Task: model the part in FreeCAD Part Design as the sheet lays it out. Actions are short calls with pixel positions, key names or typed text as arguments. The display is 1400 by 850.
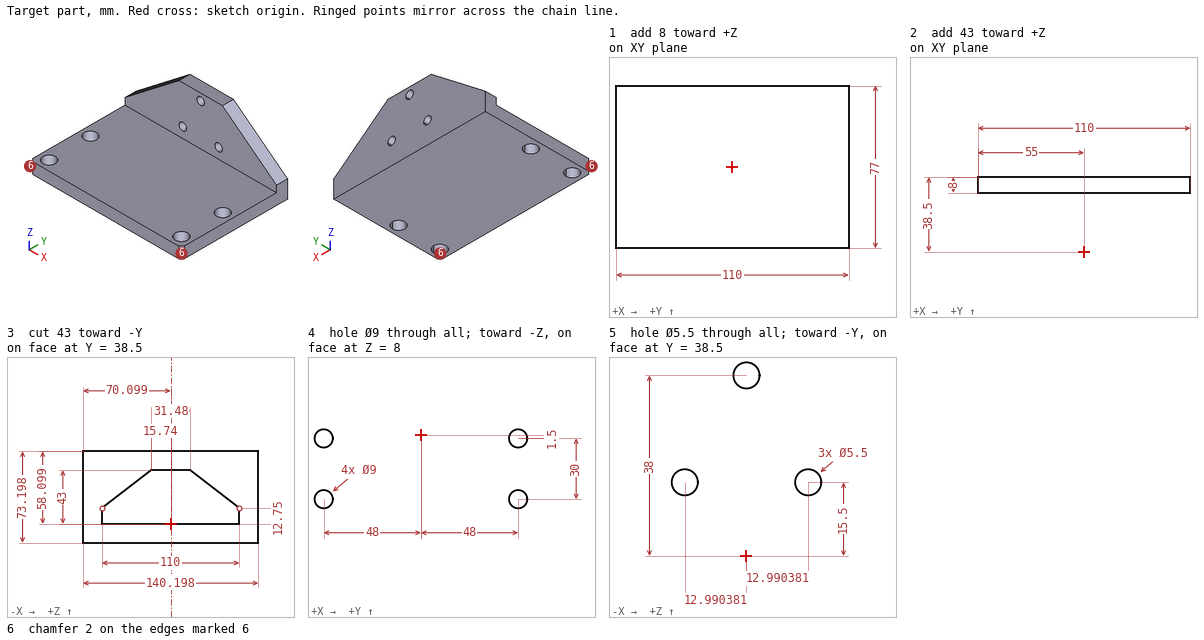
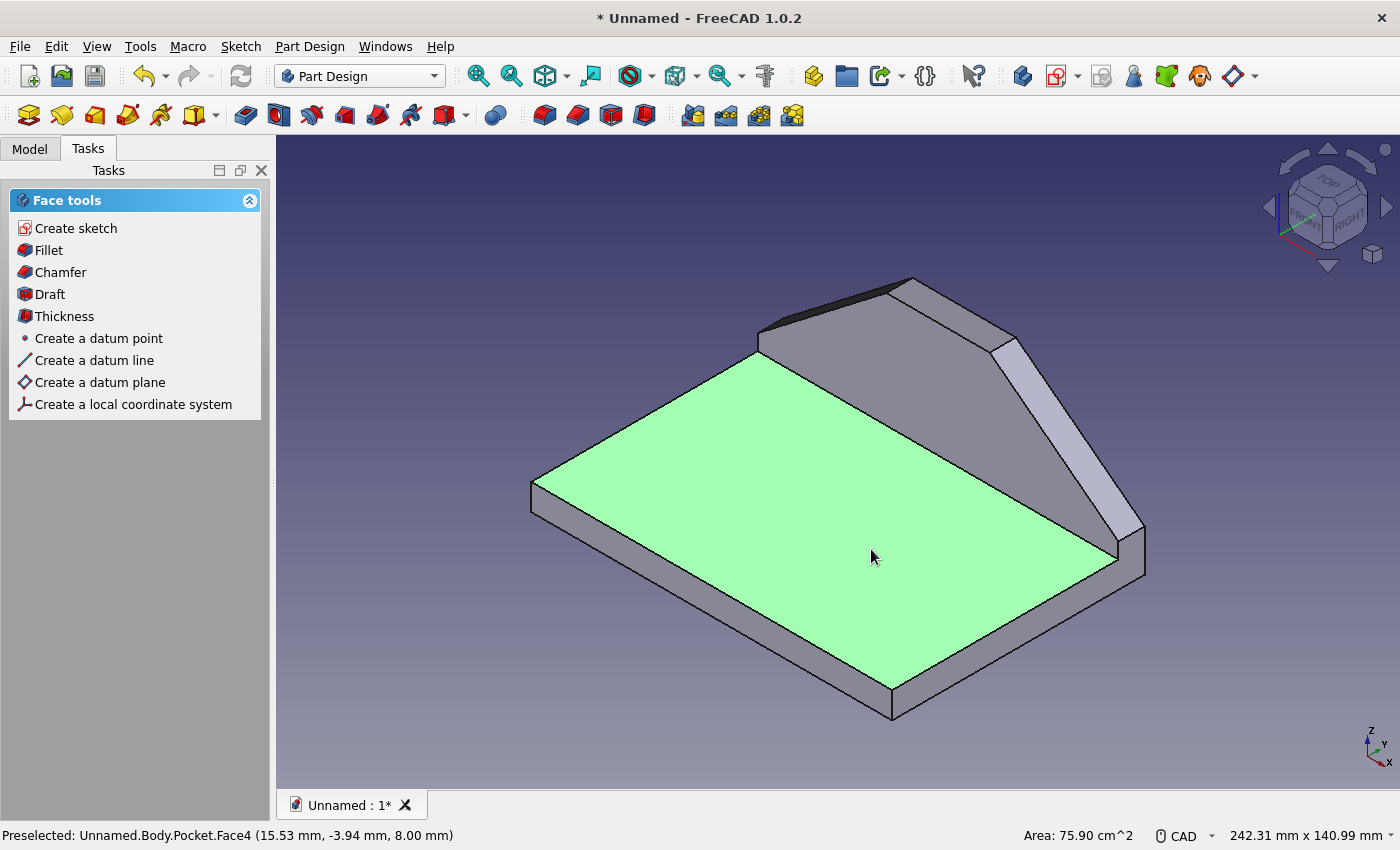
click(1056, 76)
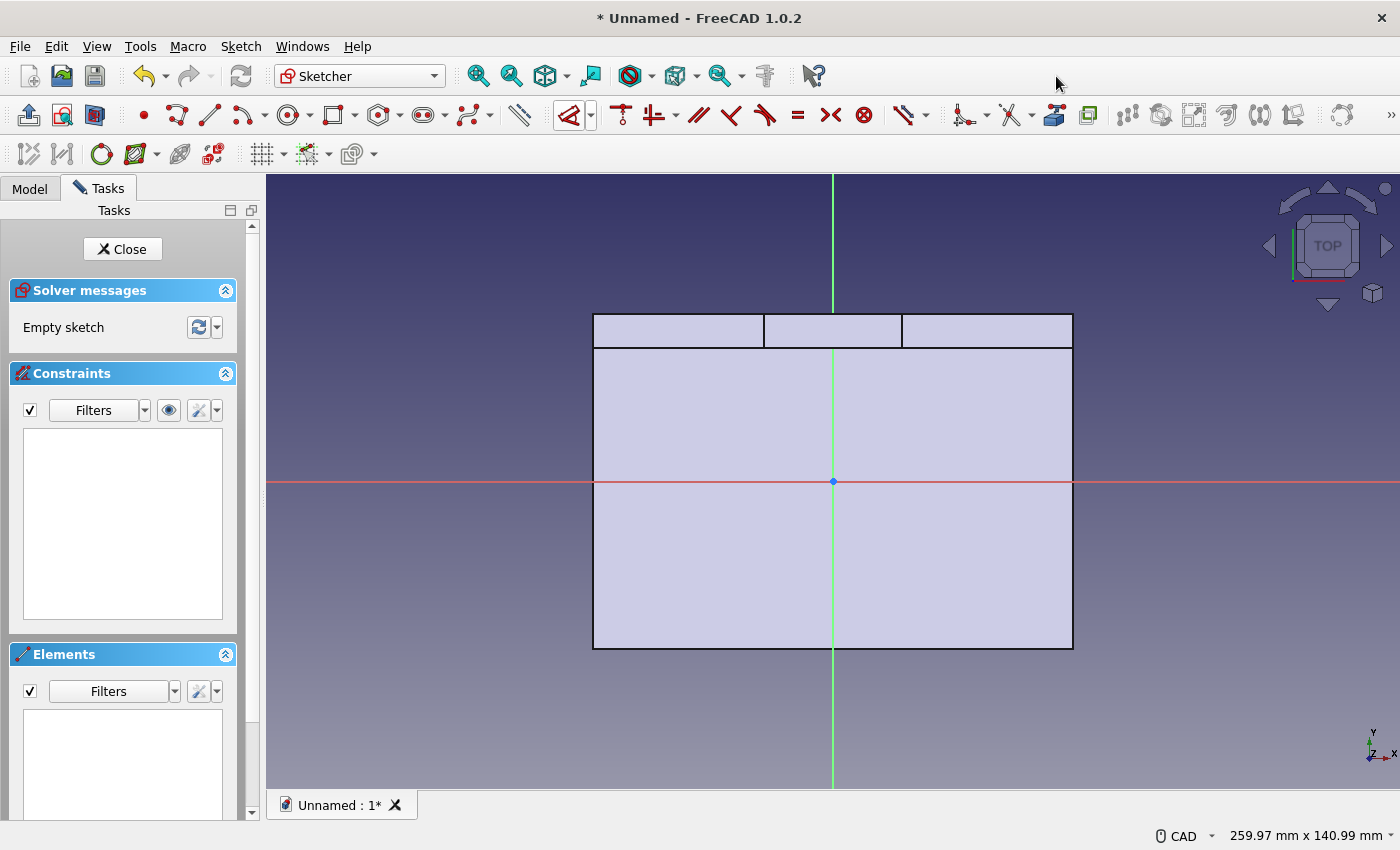
scroll(972, 700, up, 2)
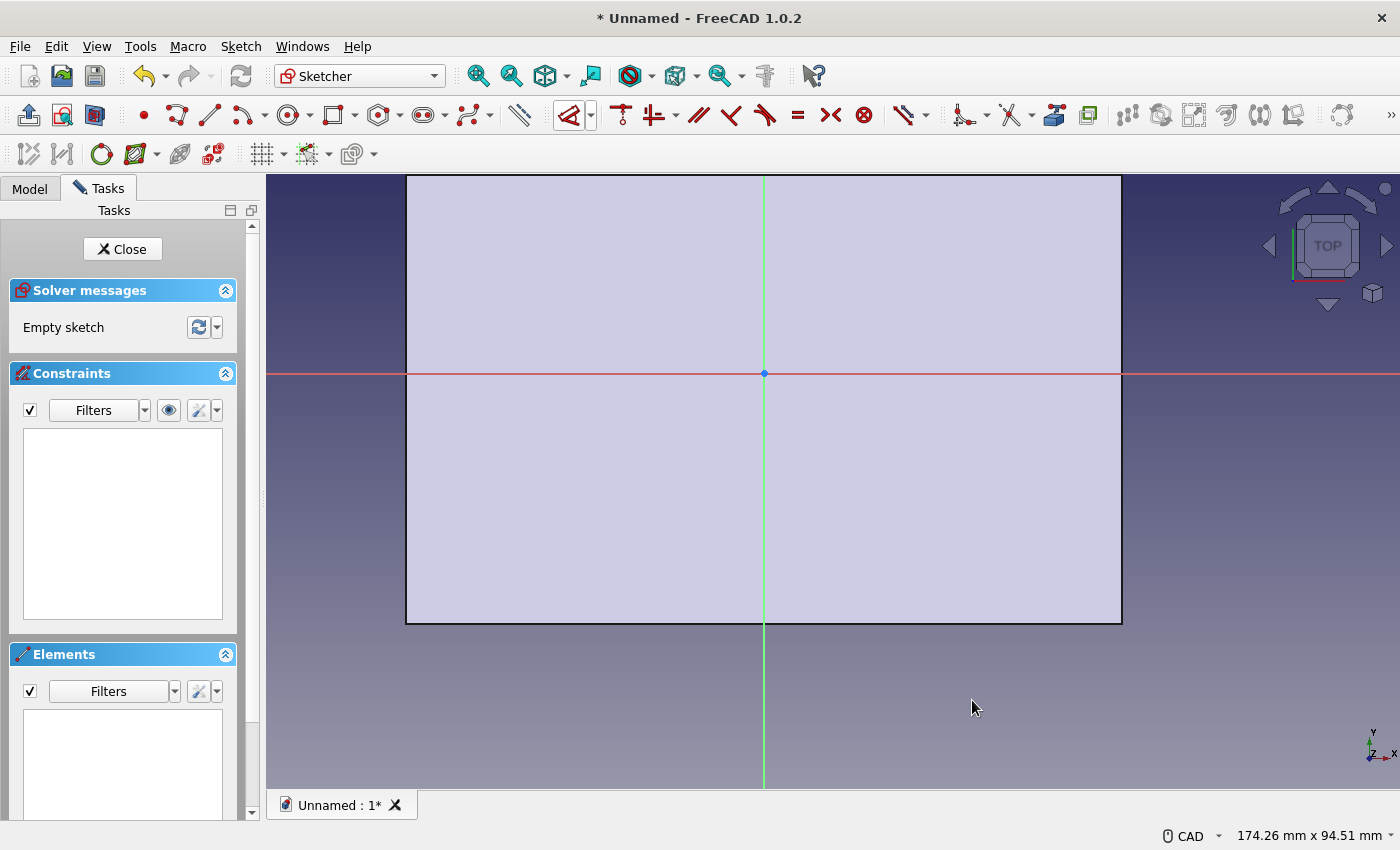
key(g)
key(c)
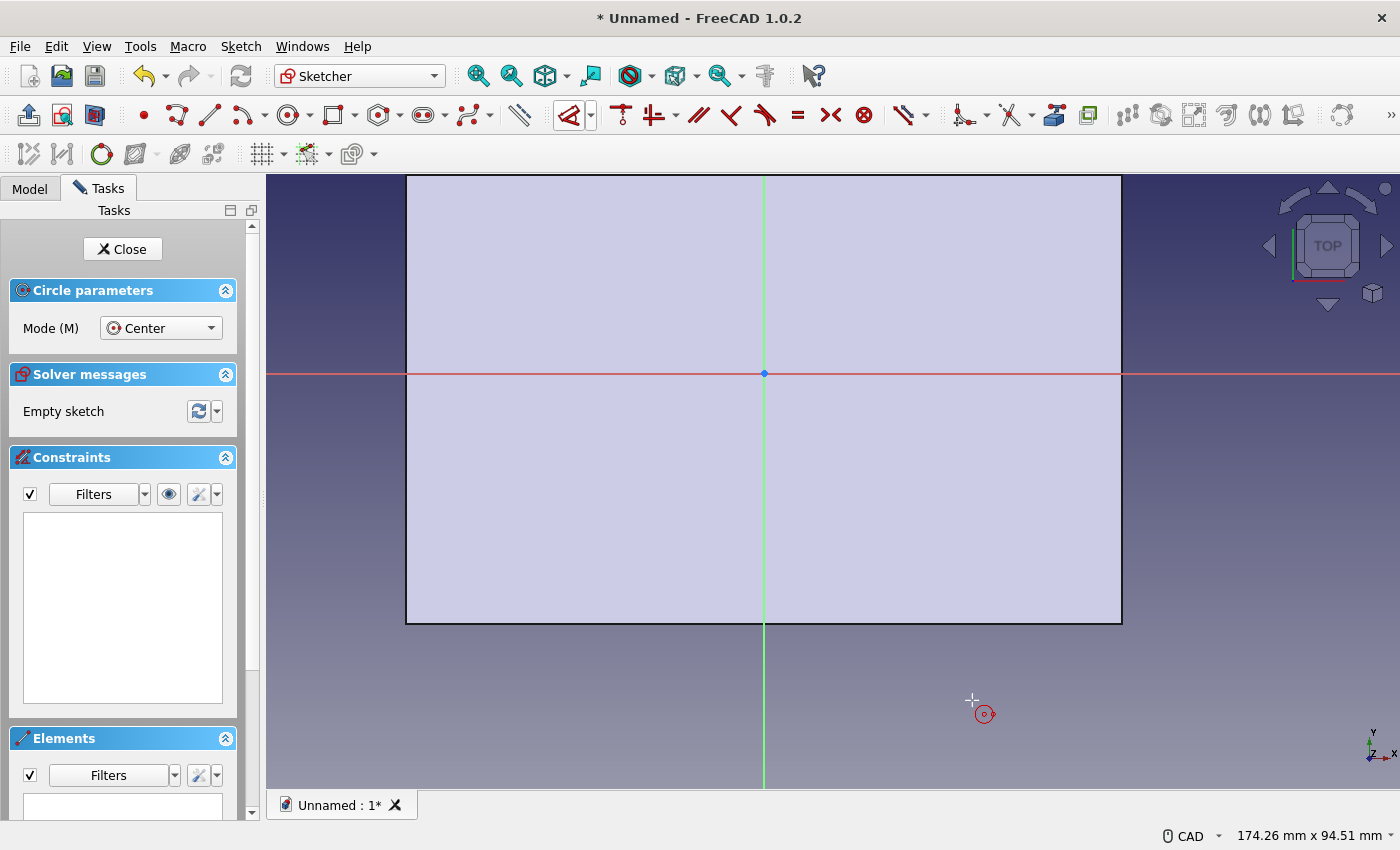
click(452, 579)
click(473, 558)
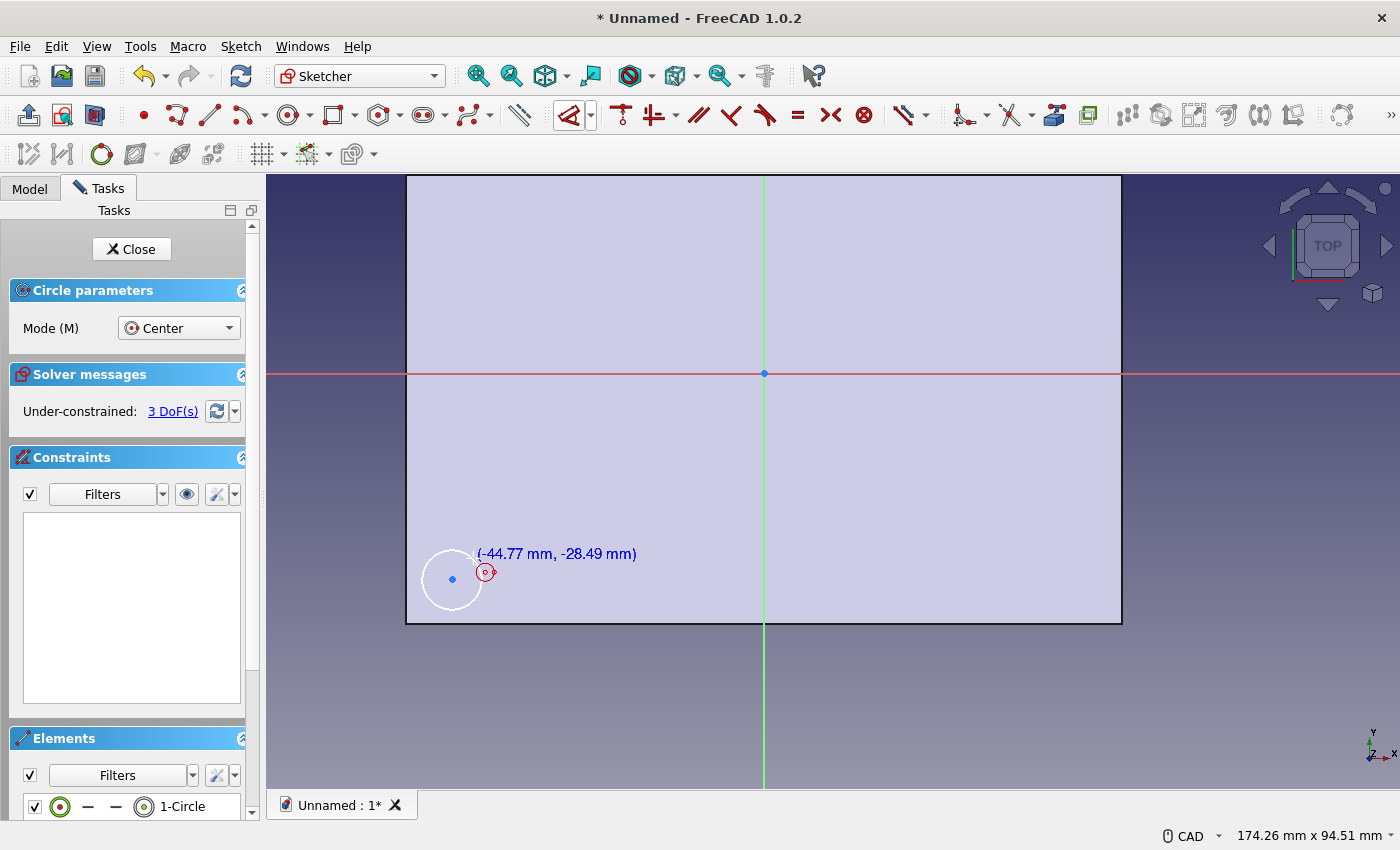
click(1077, 579)
click(1097, 558)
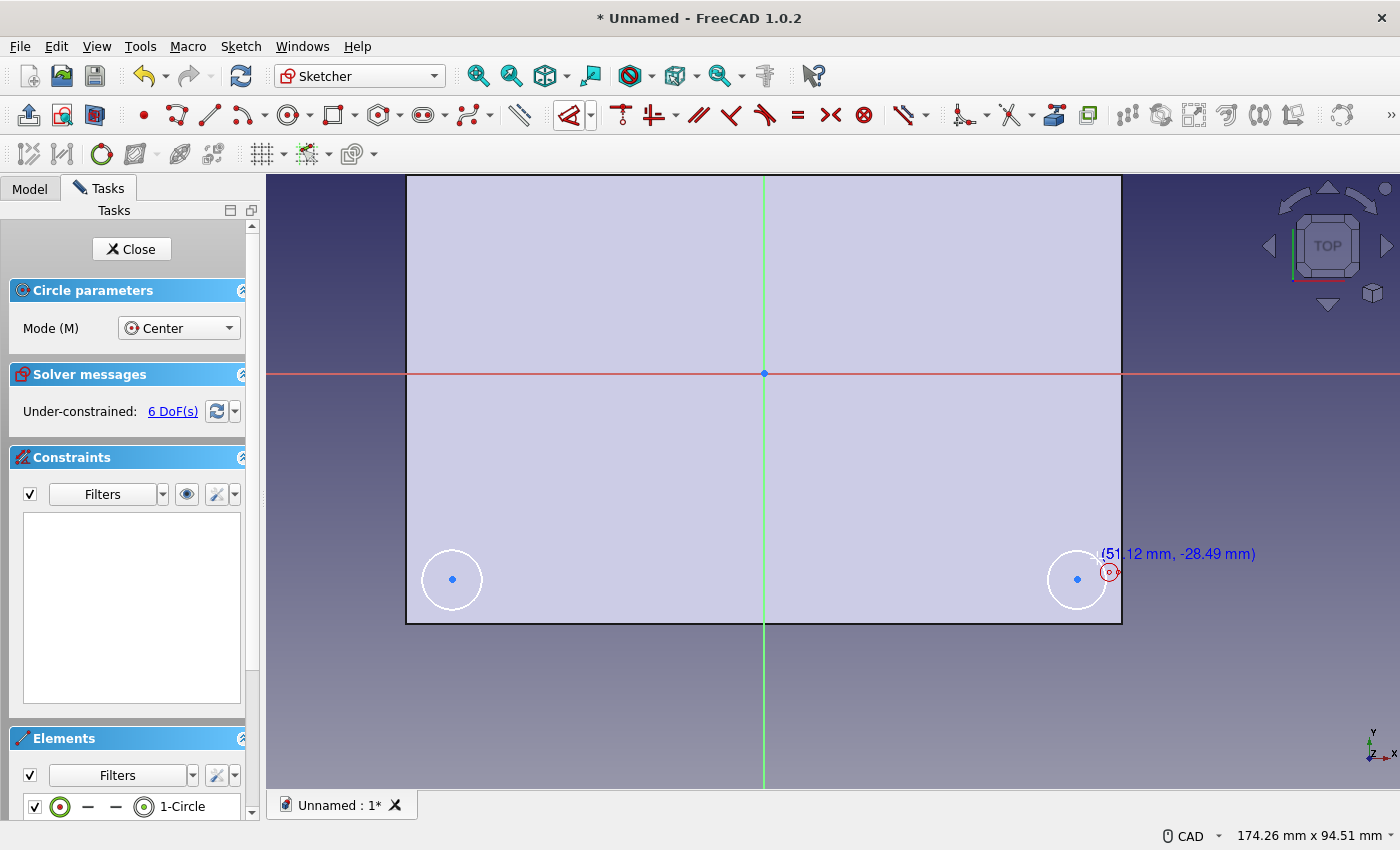
scroll(1077, 383, up, 3)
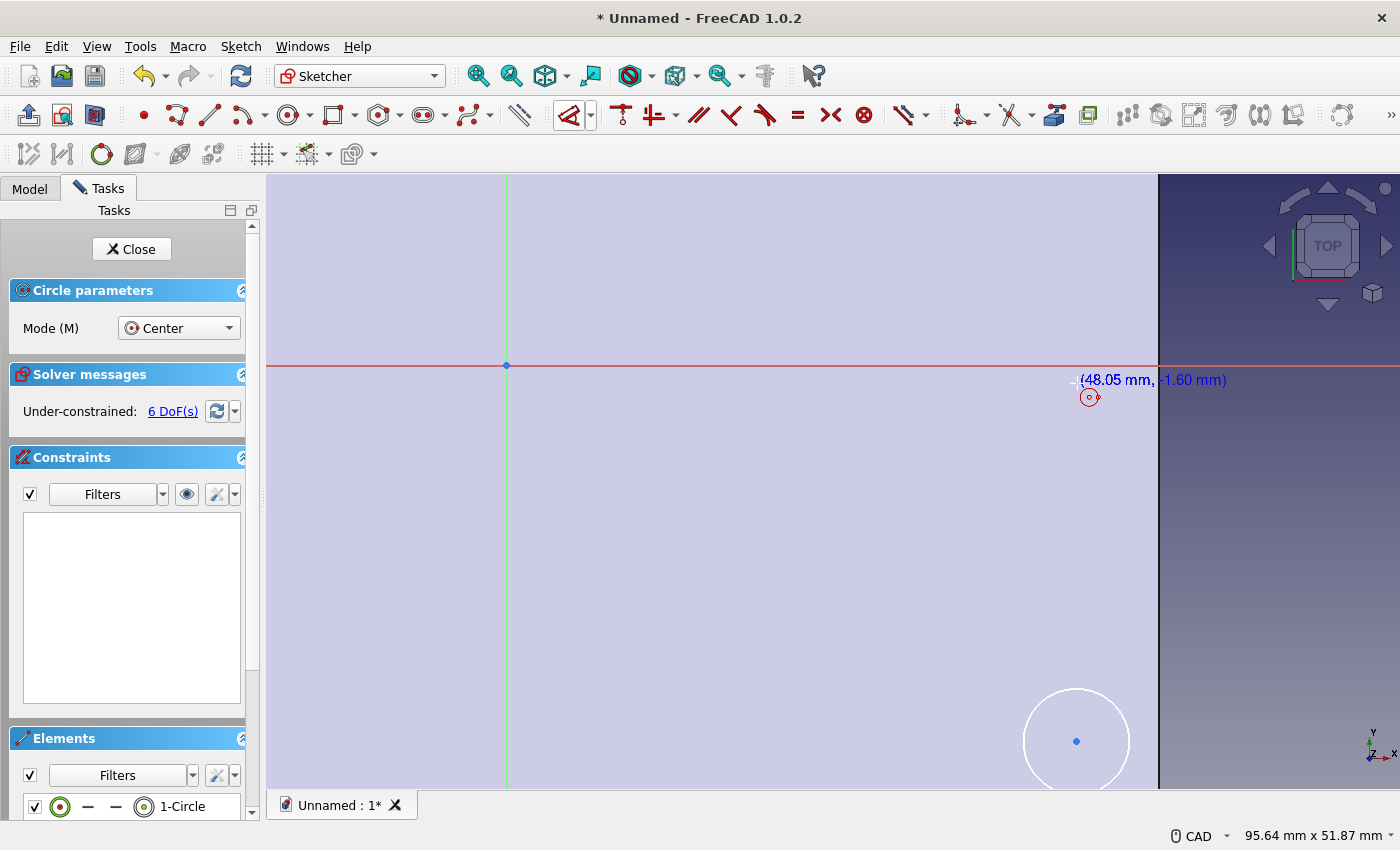
click(1076, 383)
click(1114, 346)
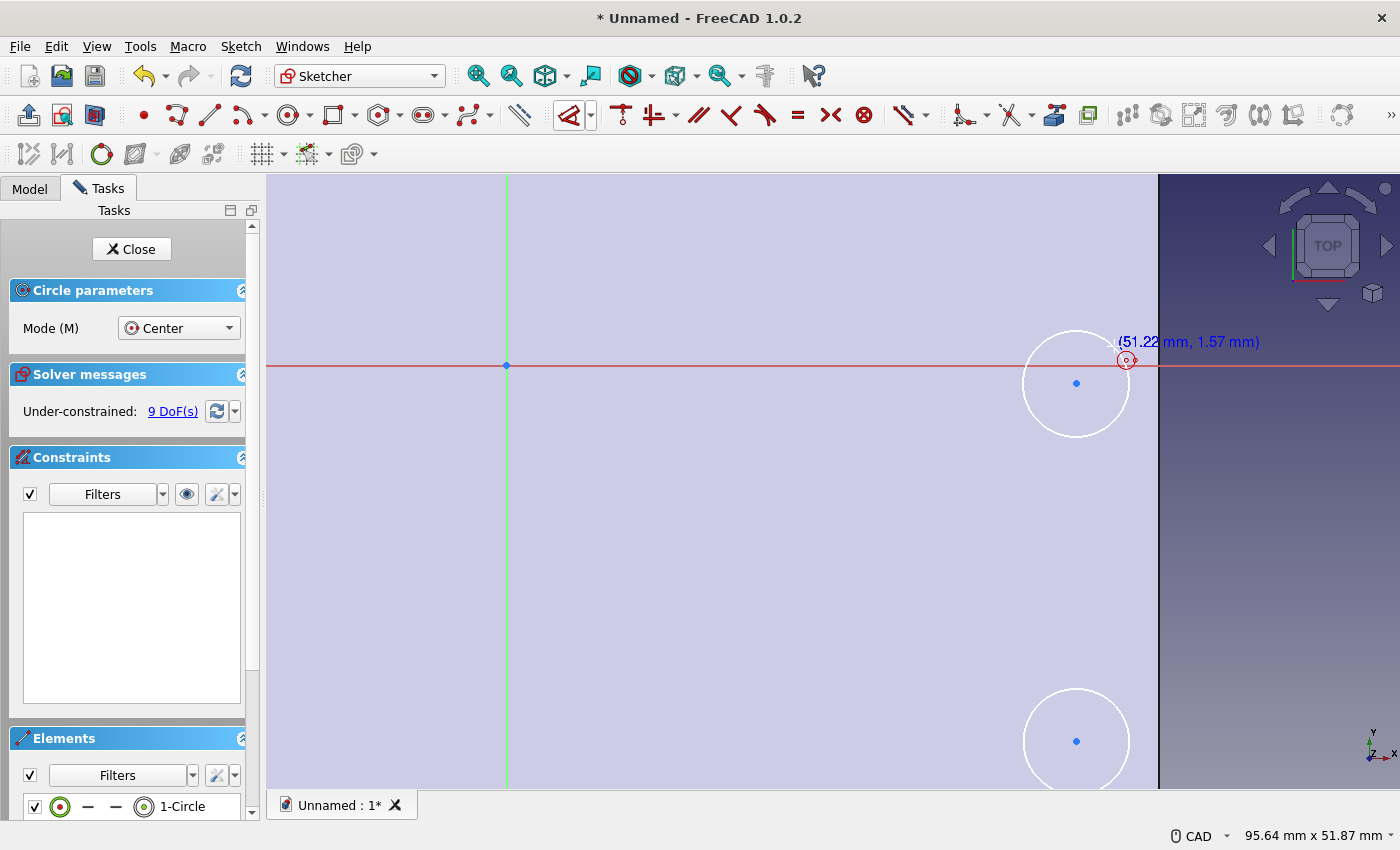
scroll(1078, 384, down, 3)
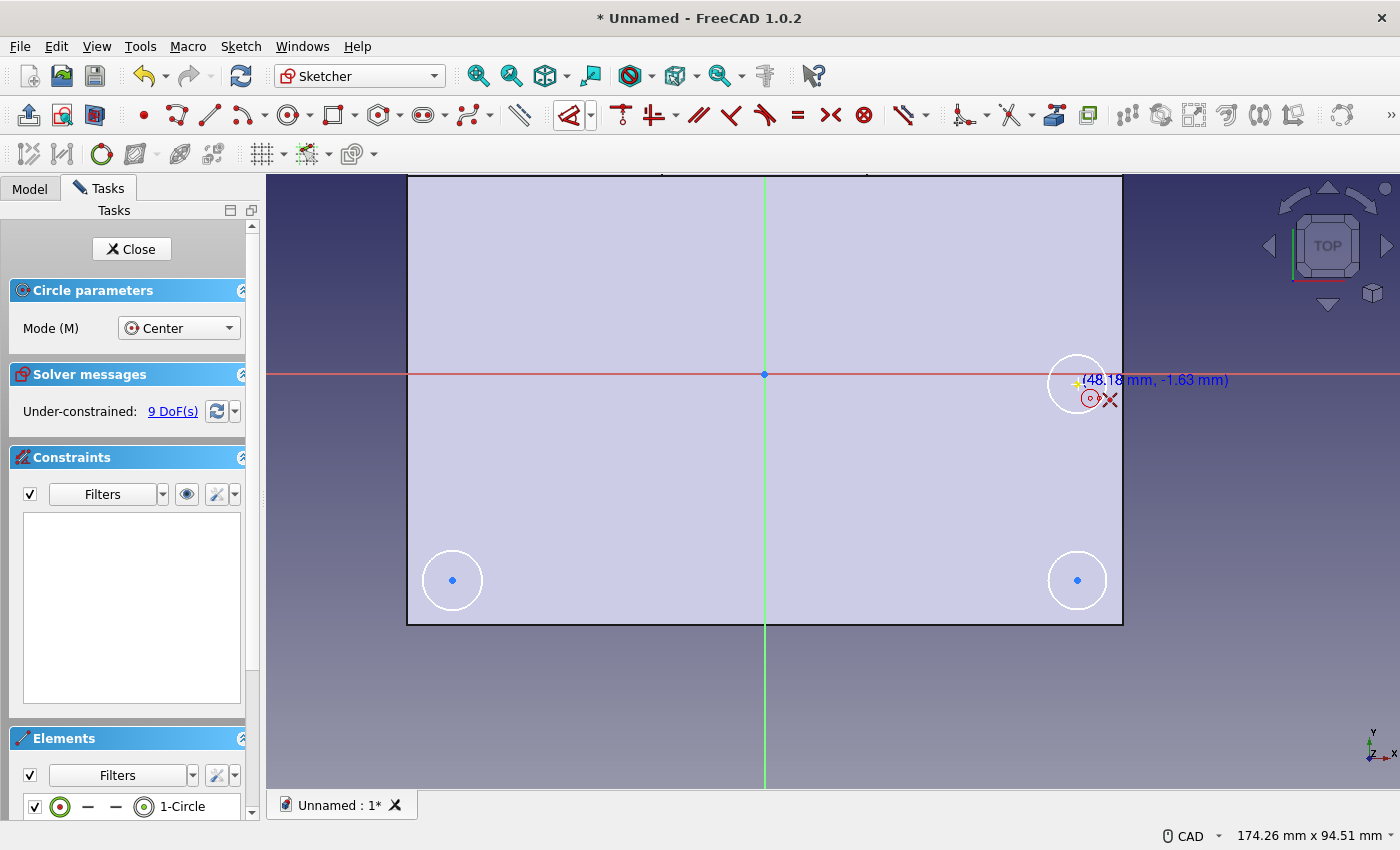
scroll(452, 384, up, 3)